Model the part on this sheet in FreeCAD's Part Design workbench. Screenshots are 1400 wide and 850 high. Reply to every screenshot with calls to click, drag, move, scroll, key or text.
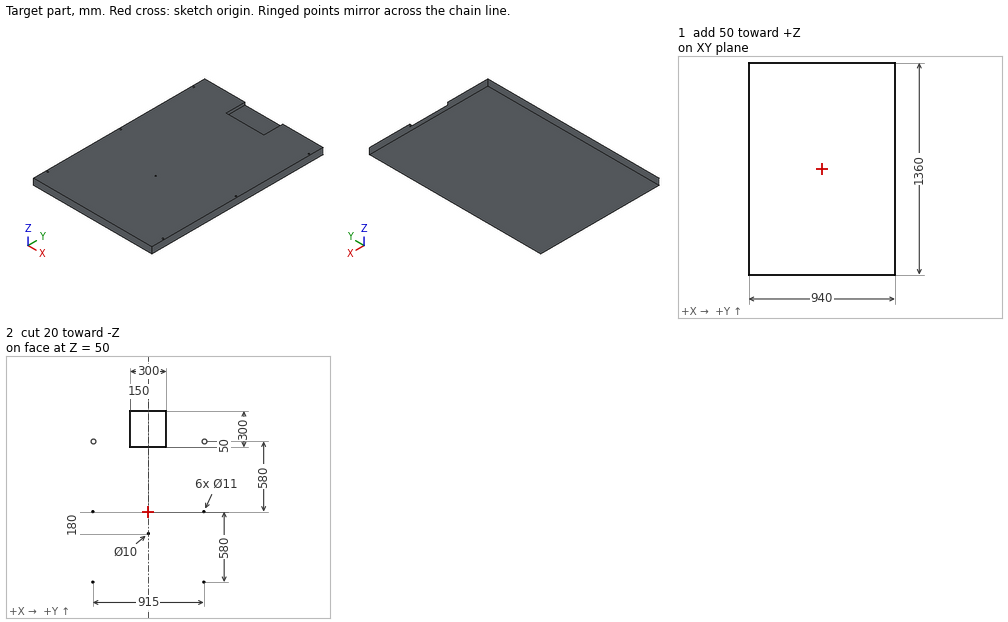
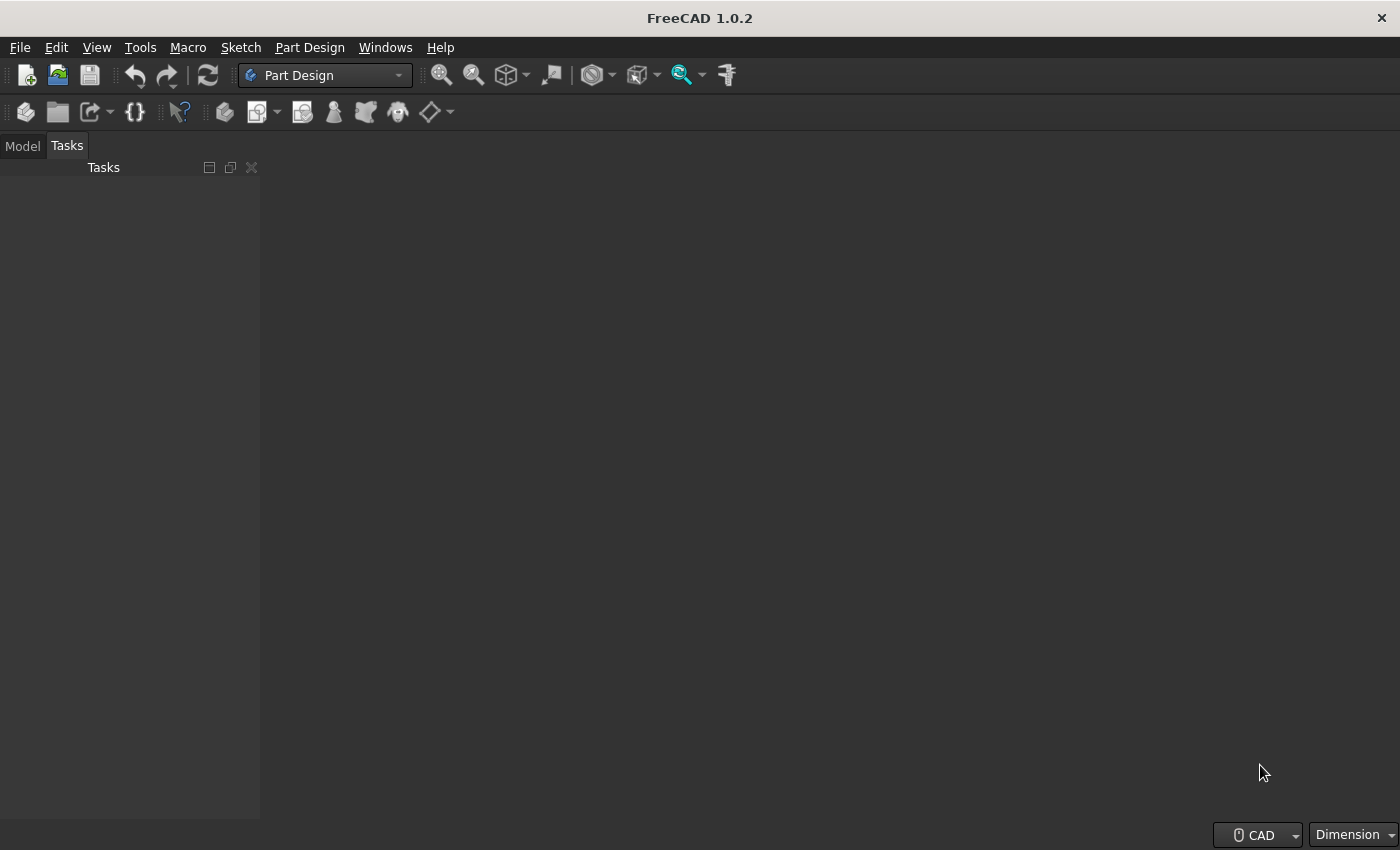
click(26, 76)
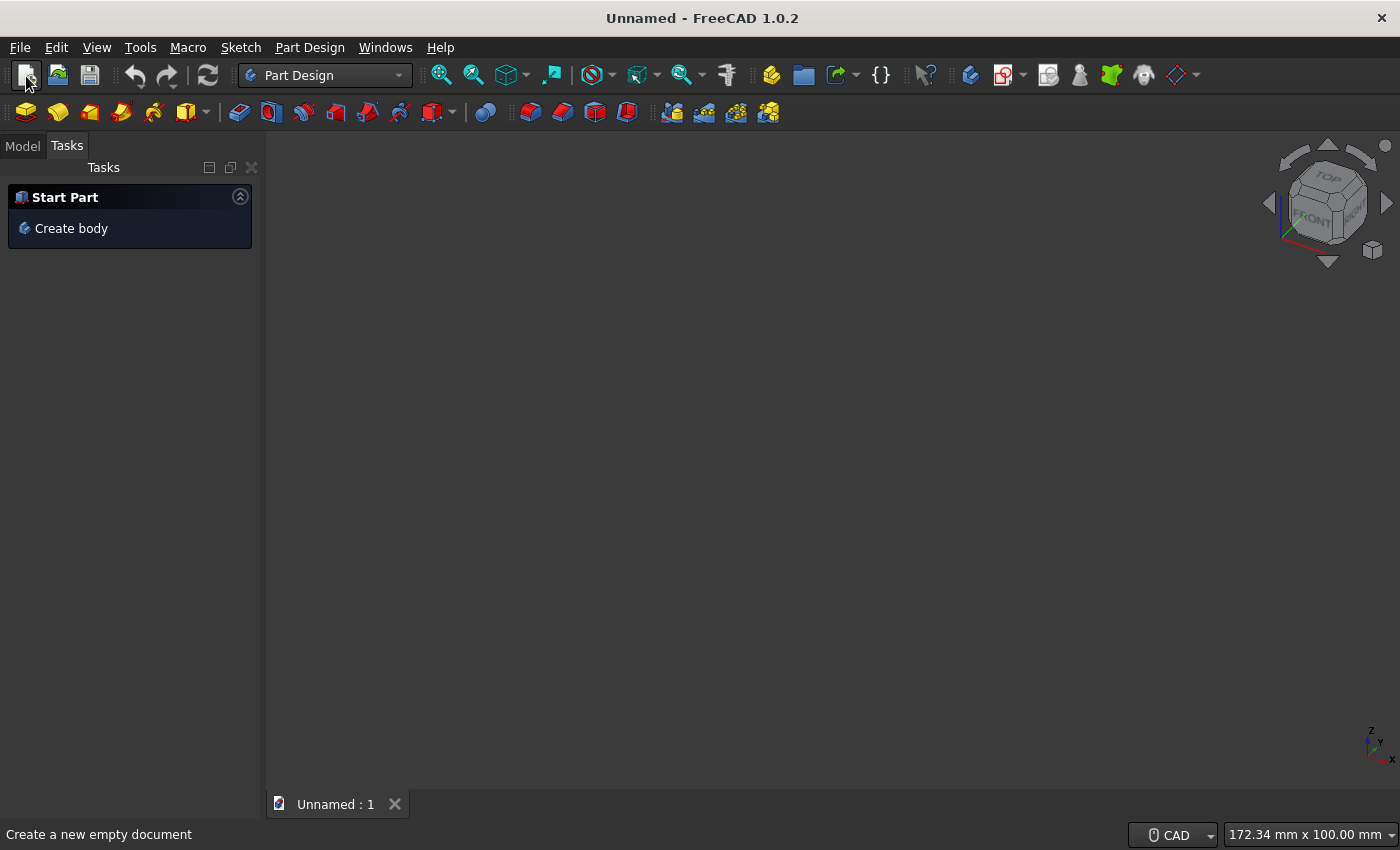
click(1004, 76)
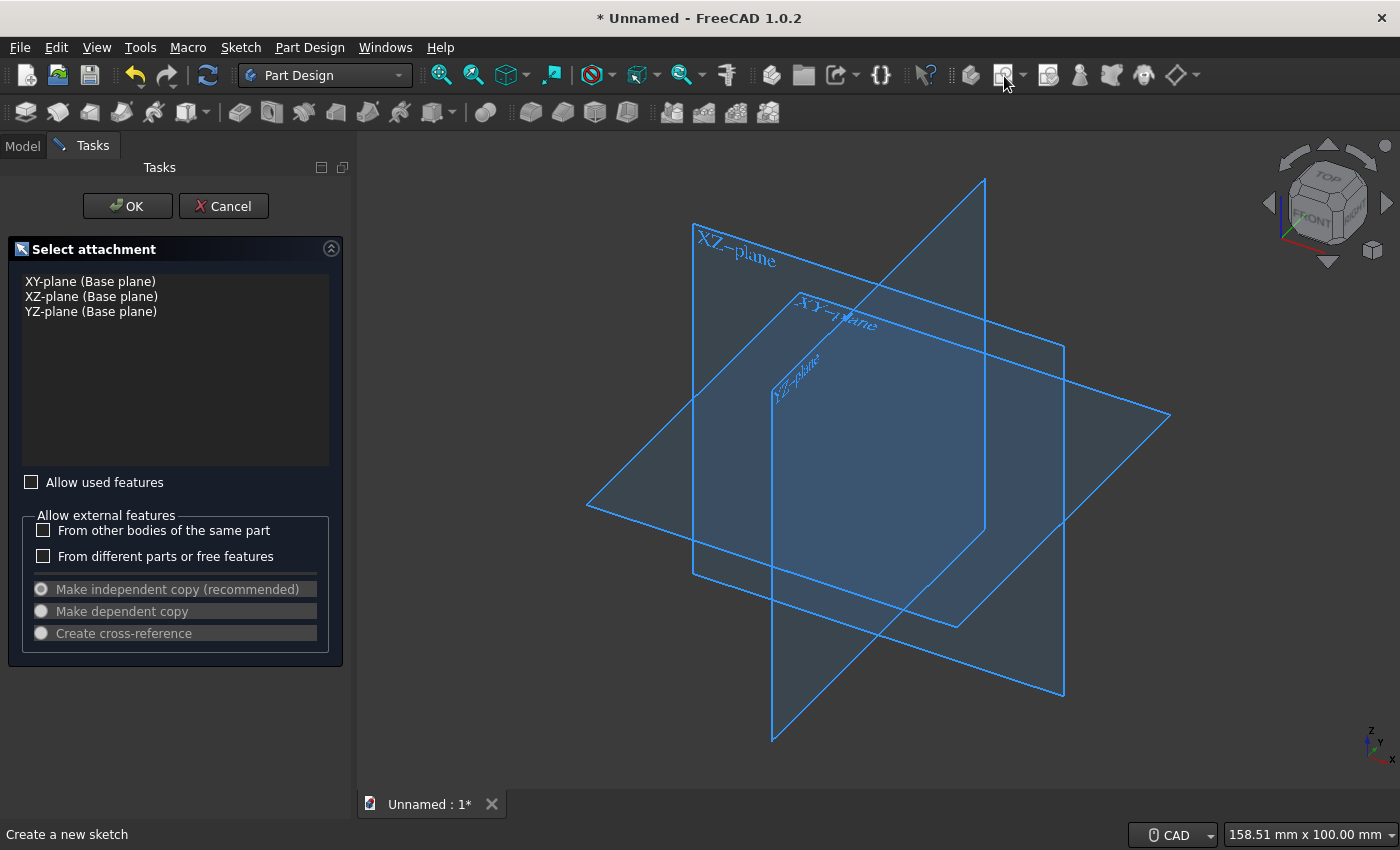
click(82, 282)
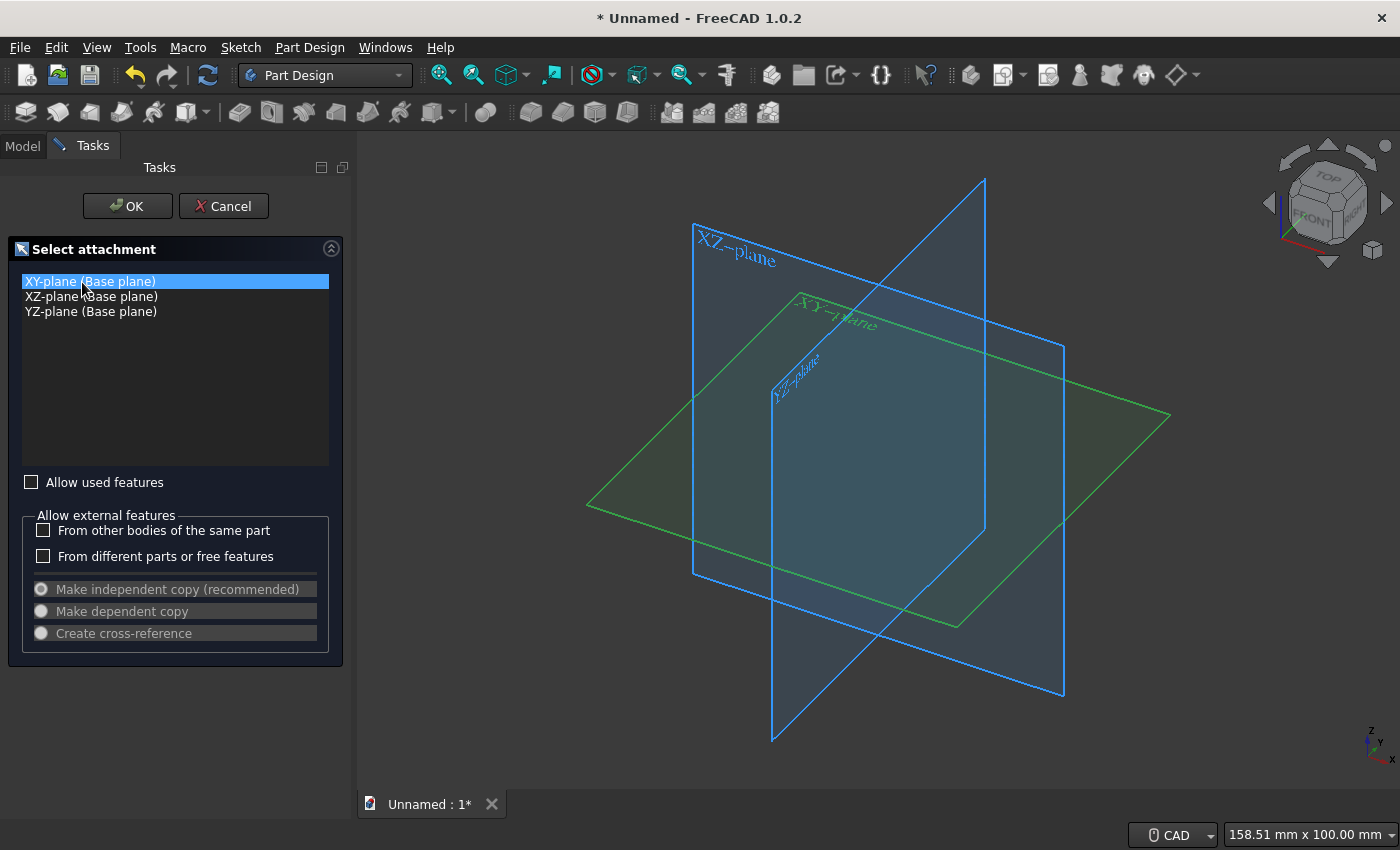
click(128, 206)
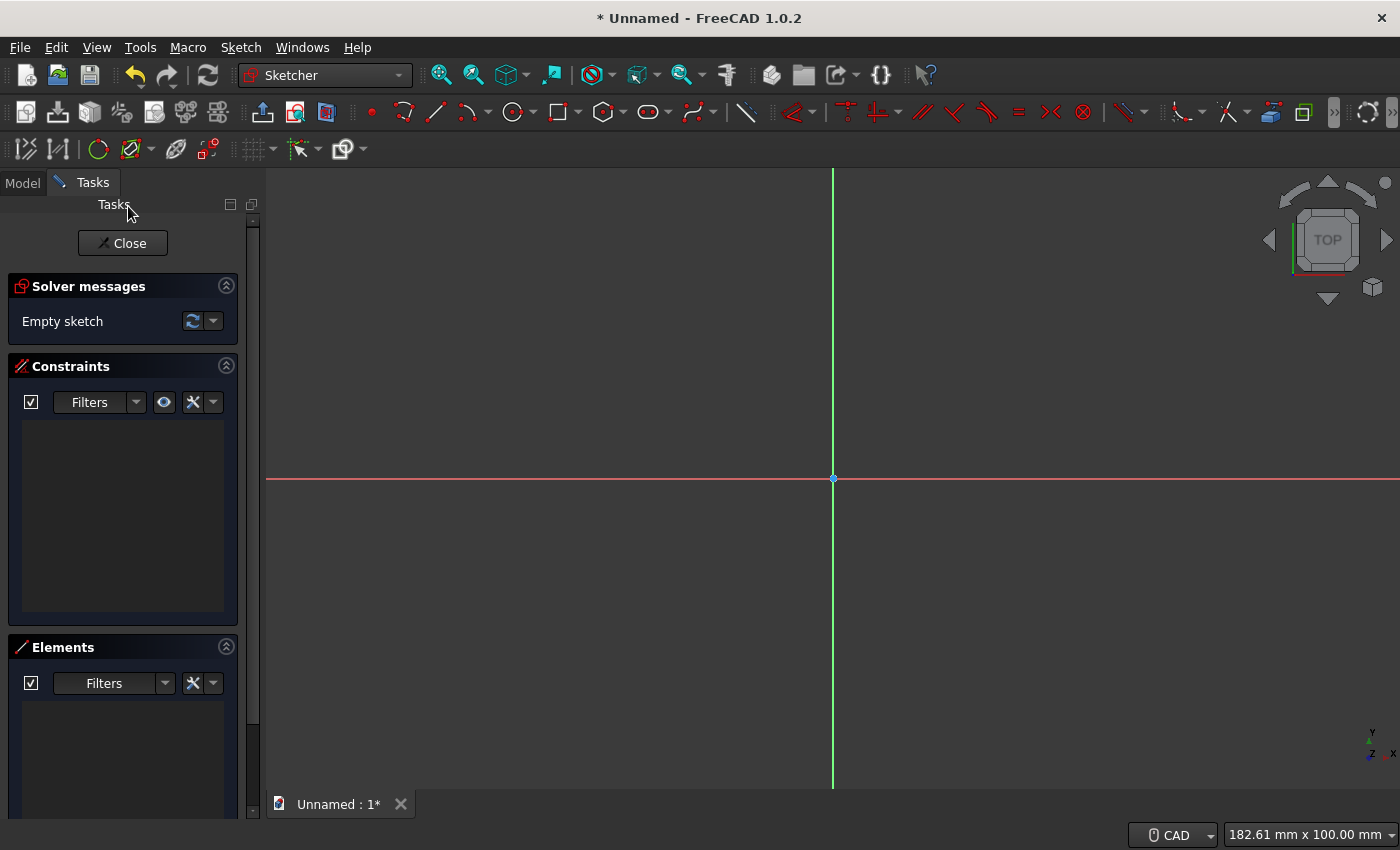
scroll(761, 478, down, 15)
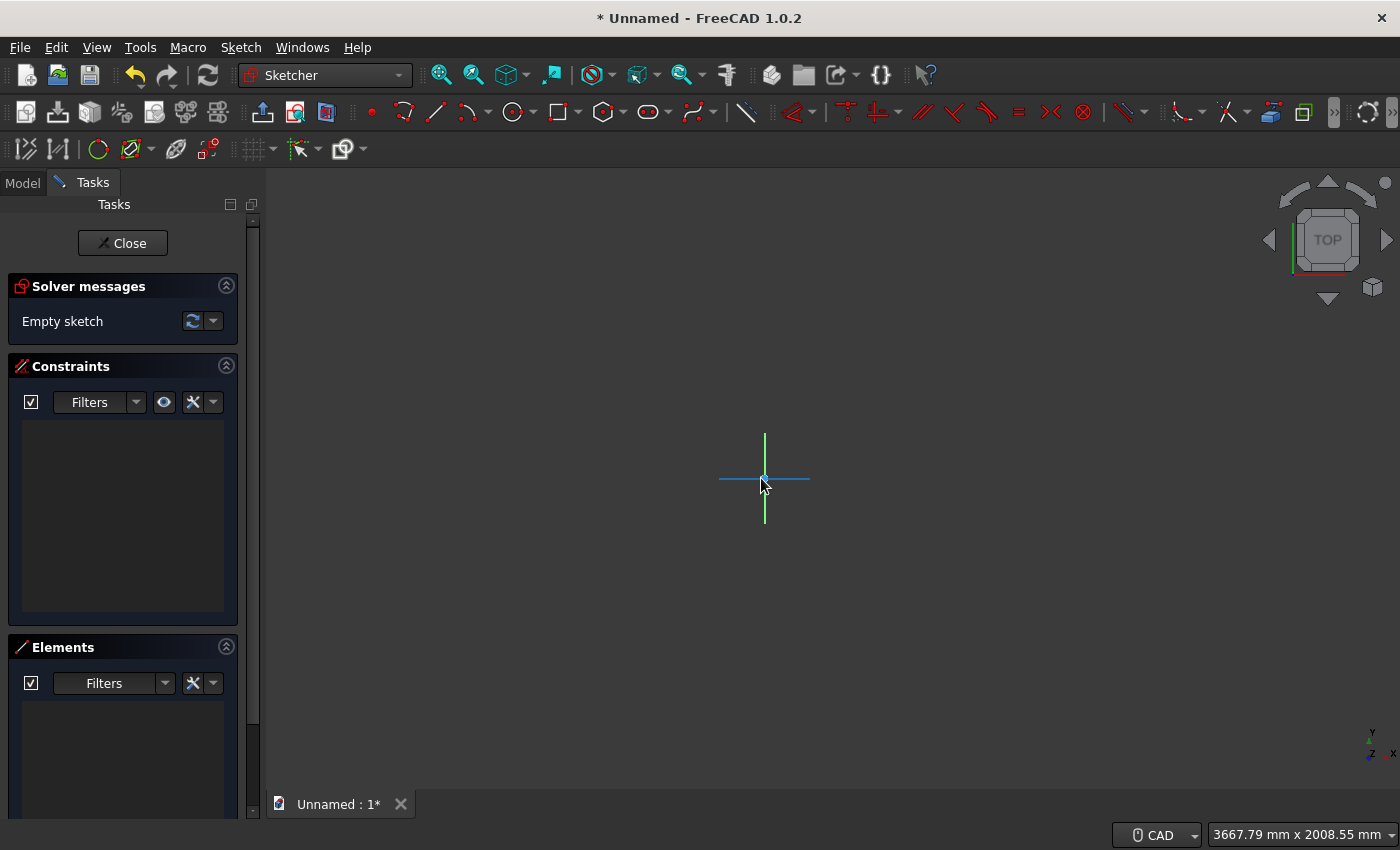
key(g)
key(v)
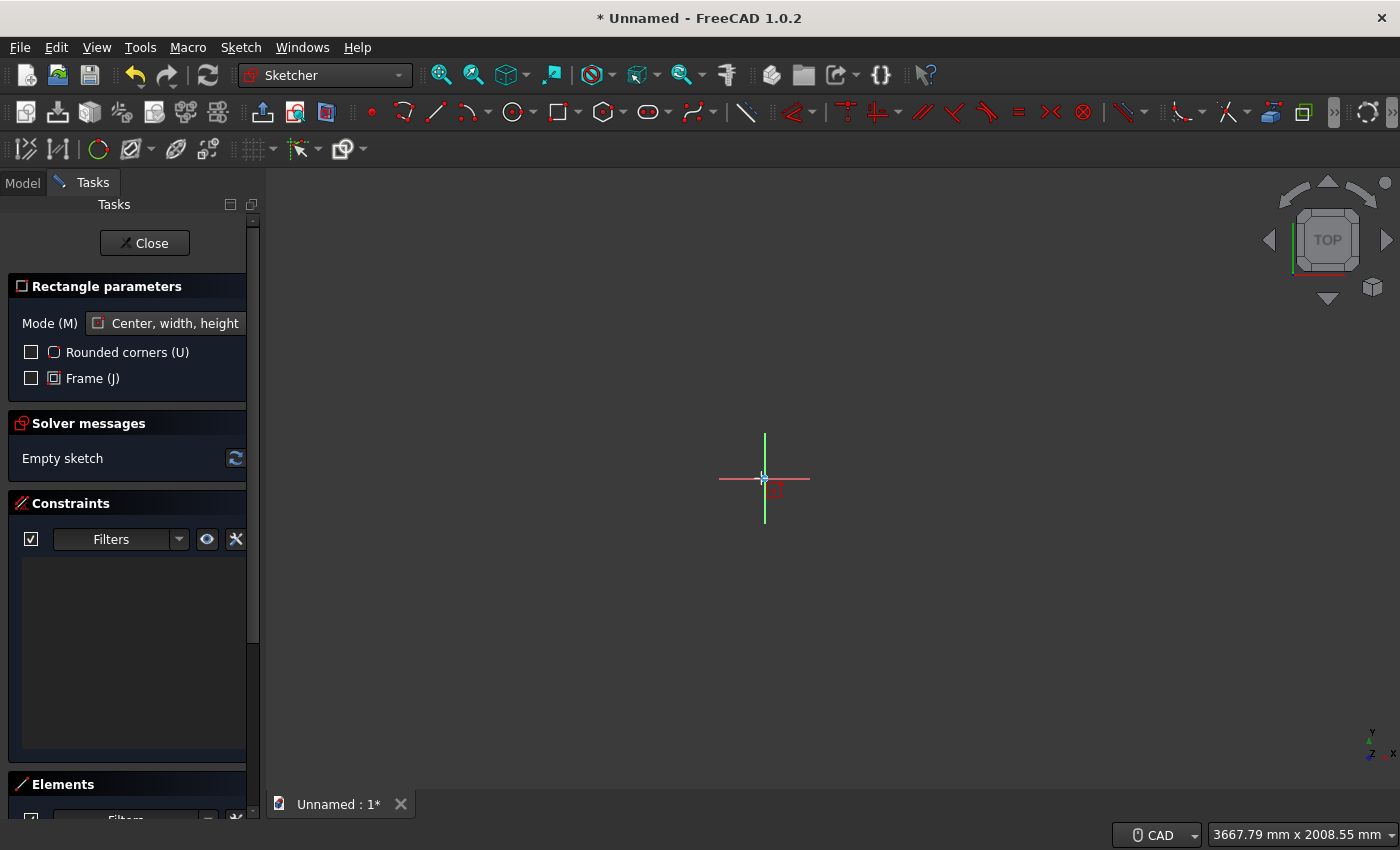
click(765, 478)
move(910, 268)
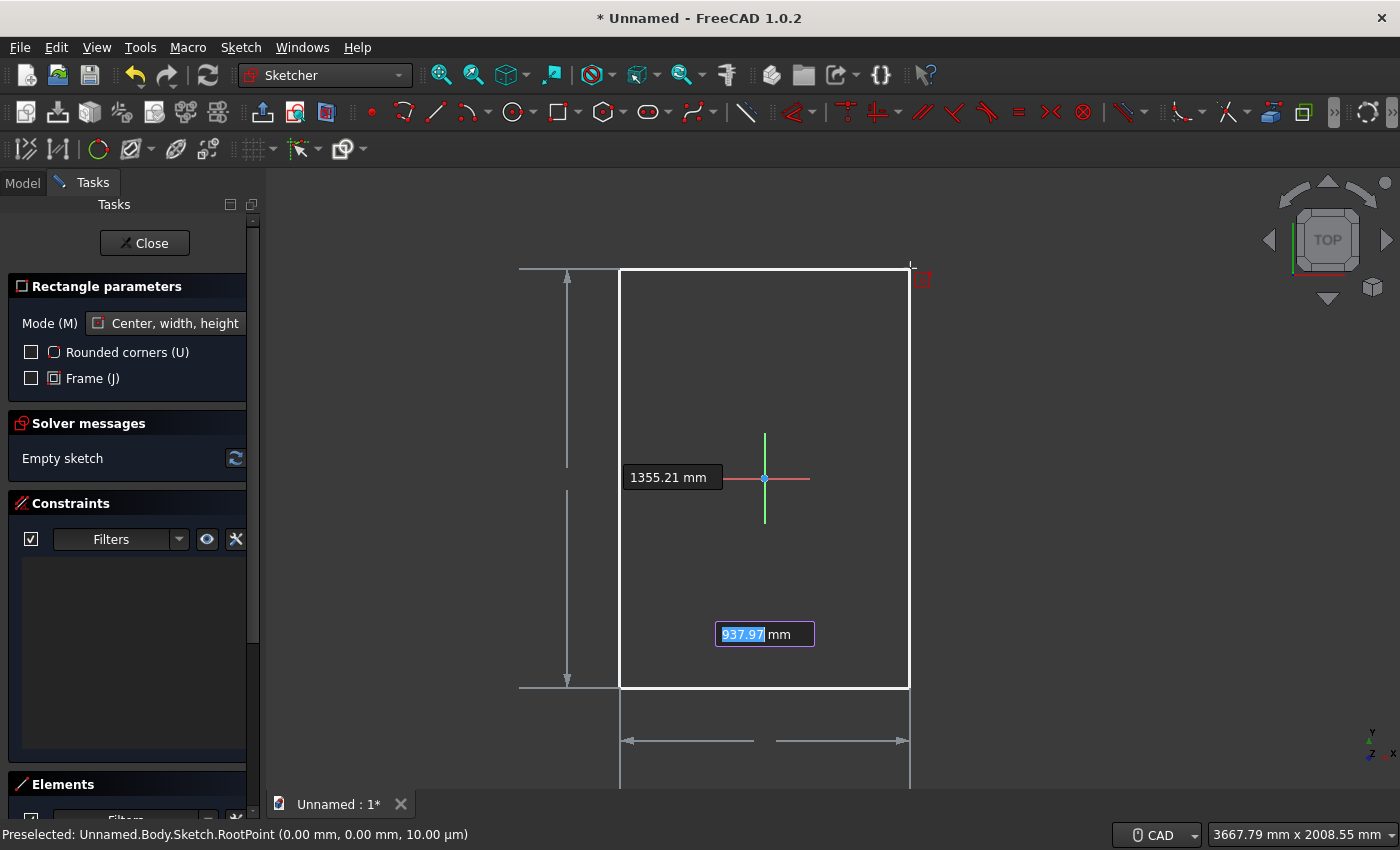
text(940)
key(Tab)
text(1360)
key(Return)
key(Escape)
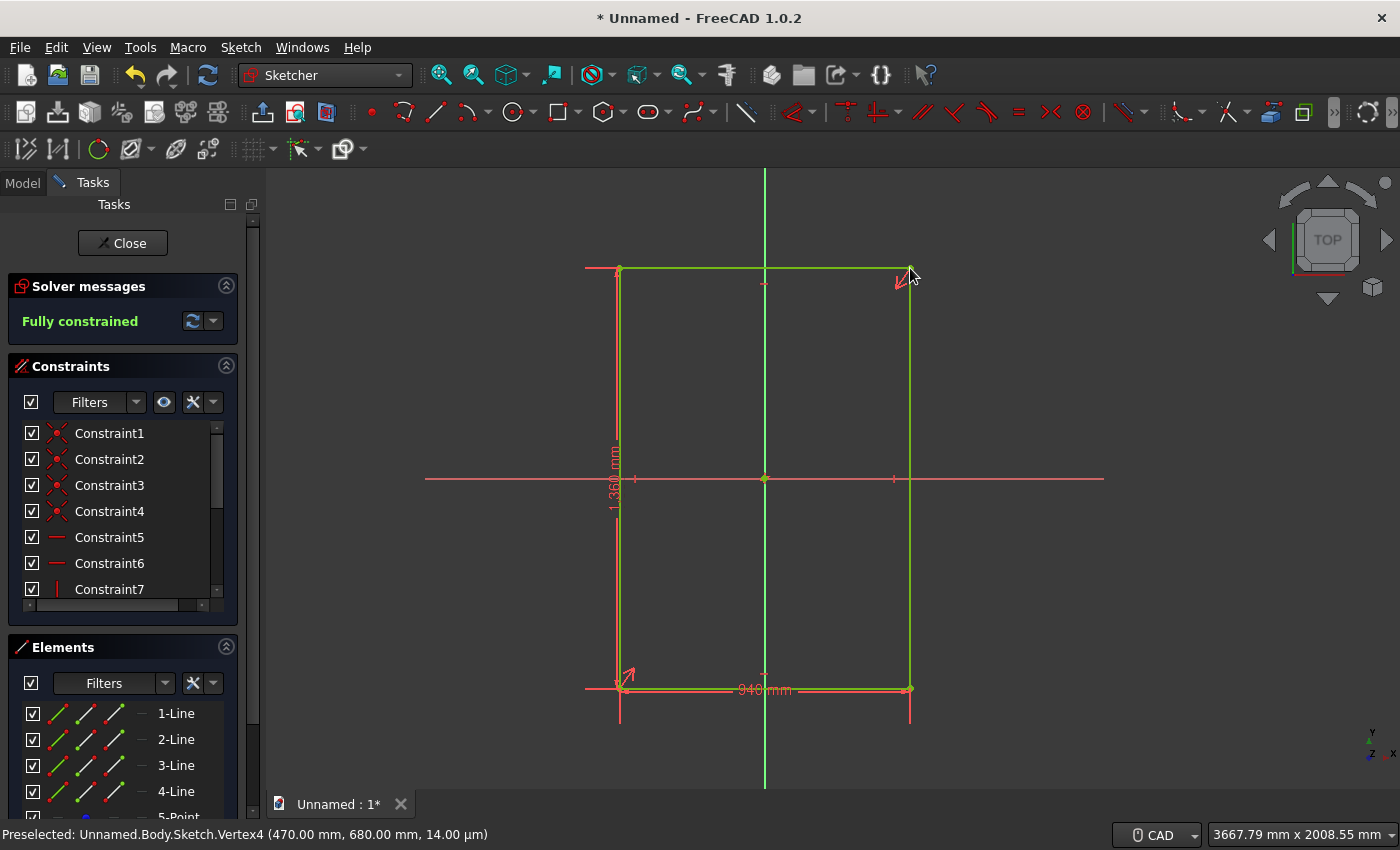
click(123, 243)